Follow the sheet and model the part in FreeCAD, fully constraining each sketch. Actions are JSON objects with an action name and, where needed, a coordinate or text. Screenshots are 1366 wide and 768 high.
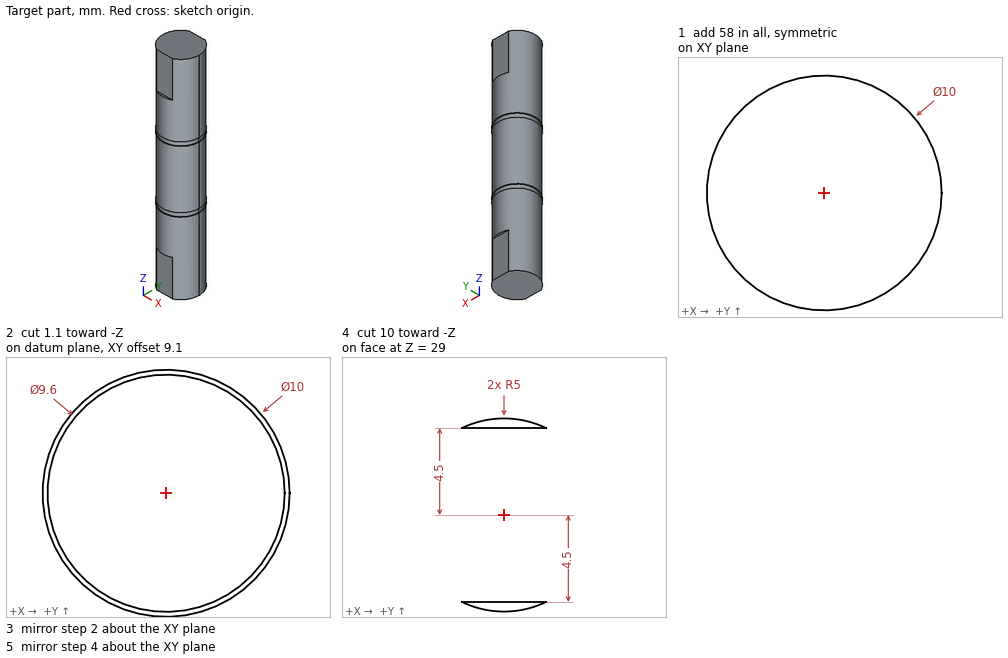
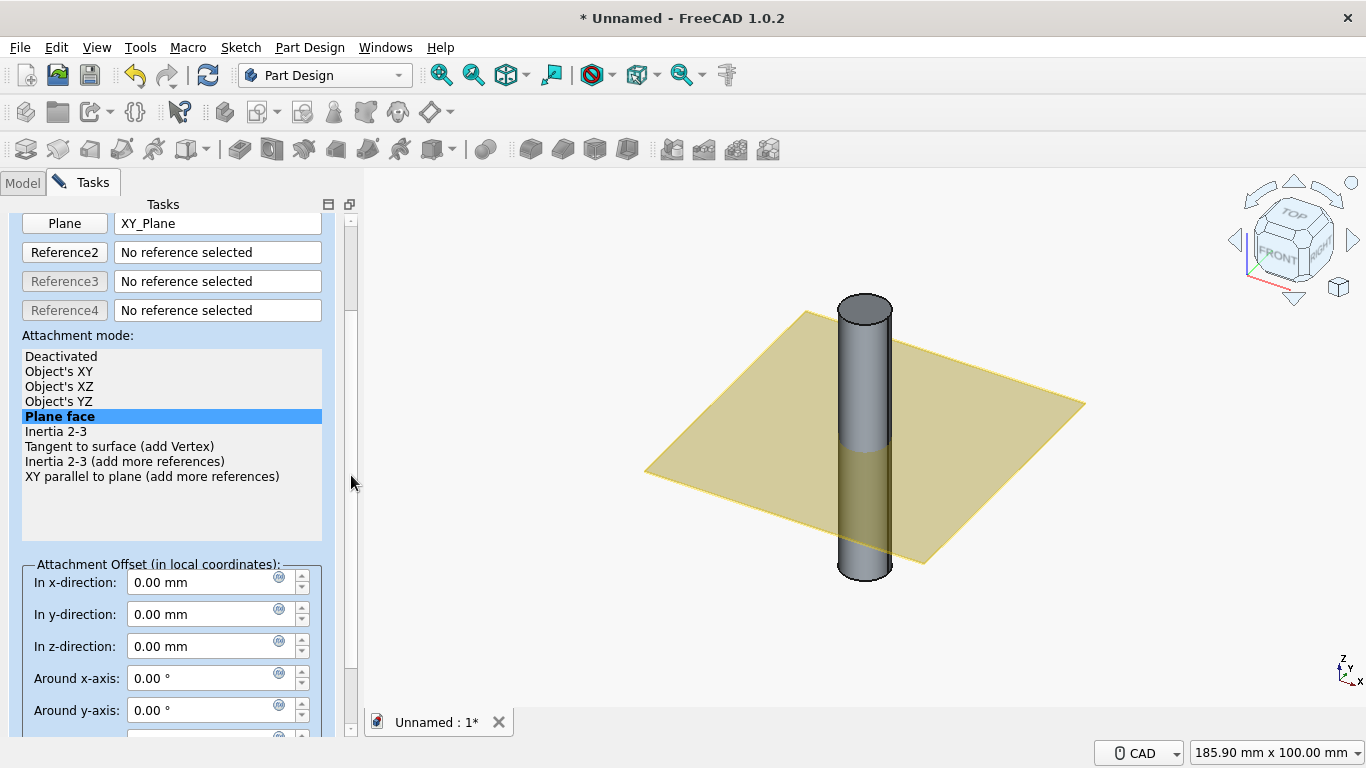
{"action": "triple_click", "coordinate": [210, 646]}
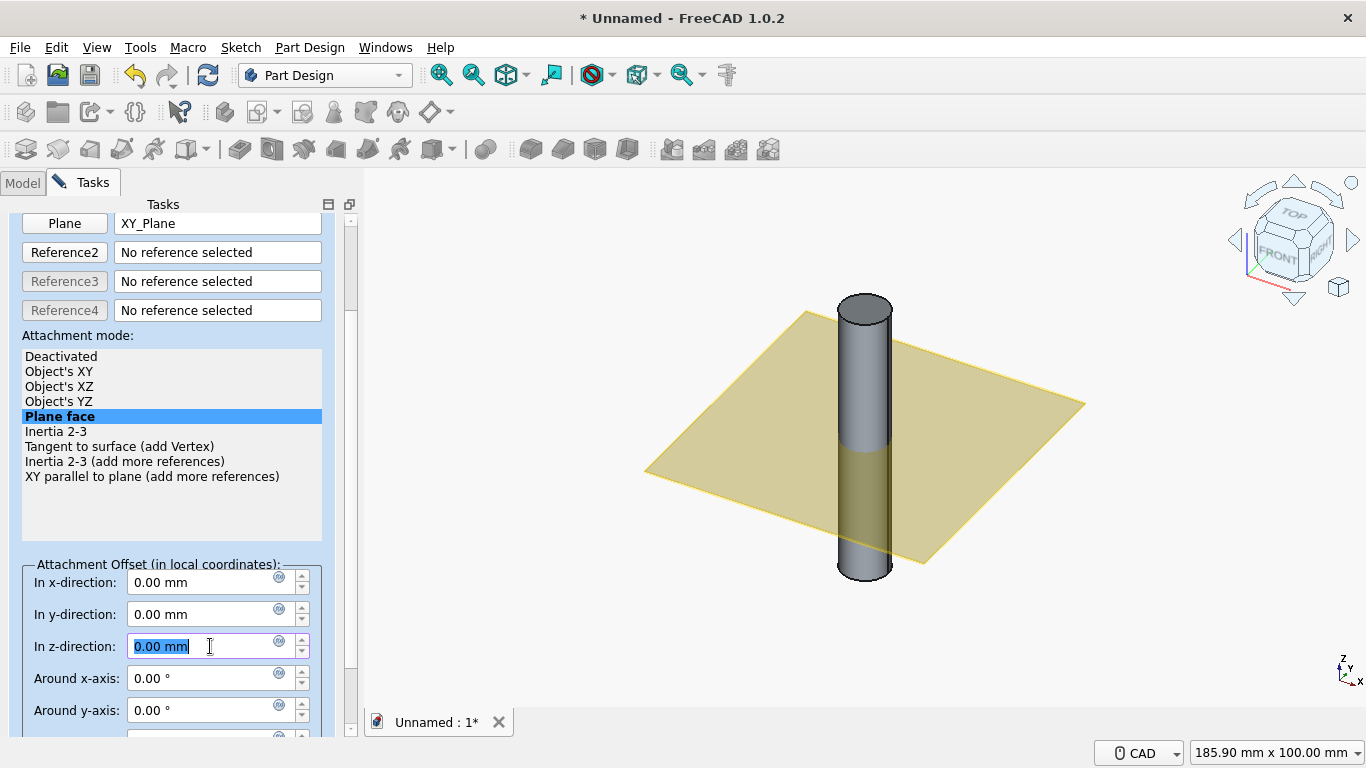
{"action": "type", "text": "9.1"}
{"action": "key", "text": "Tab"}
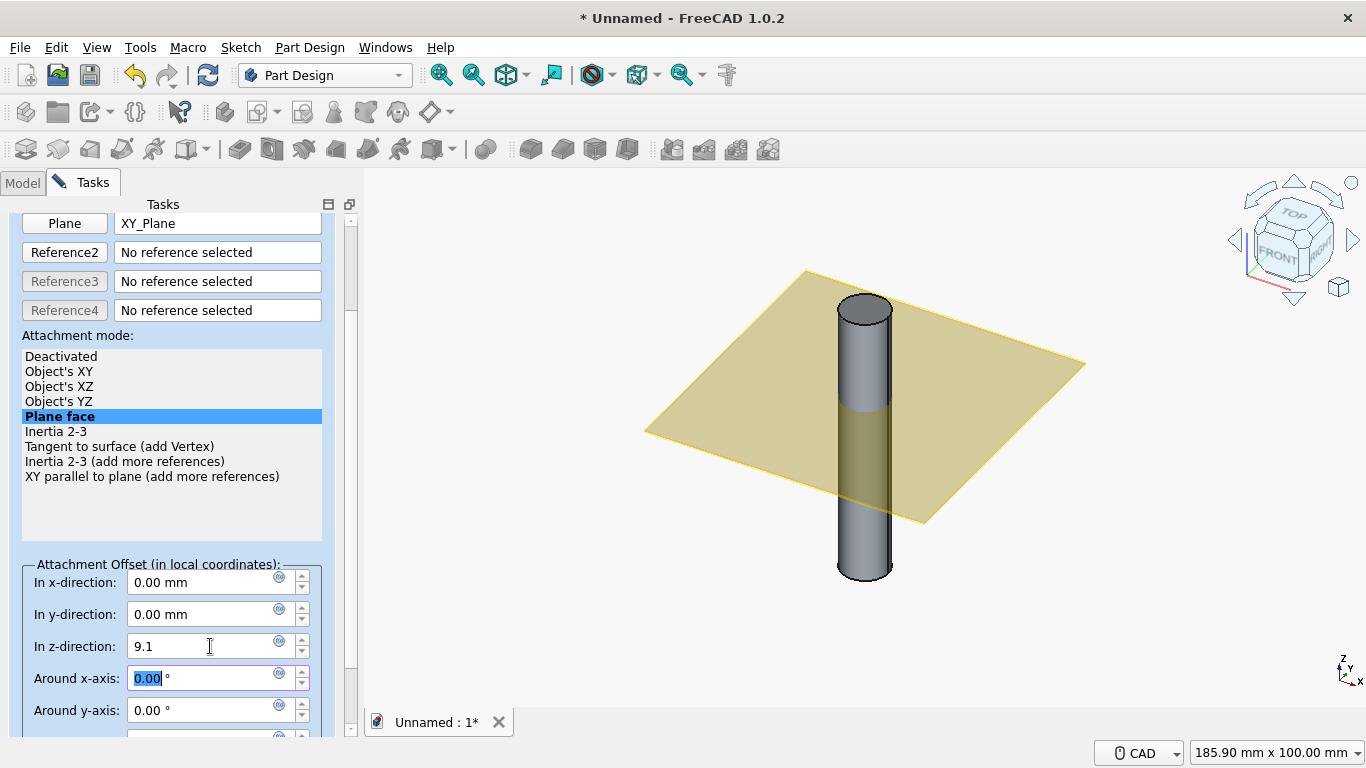
{"action": "scroll", "coordinate": [351, 475], "scroll_direction": "up", "scroll_amount": 3}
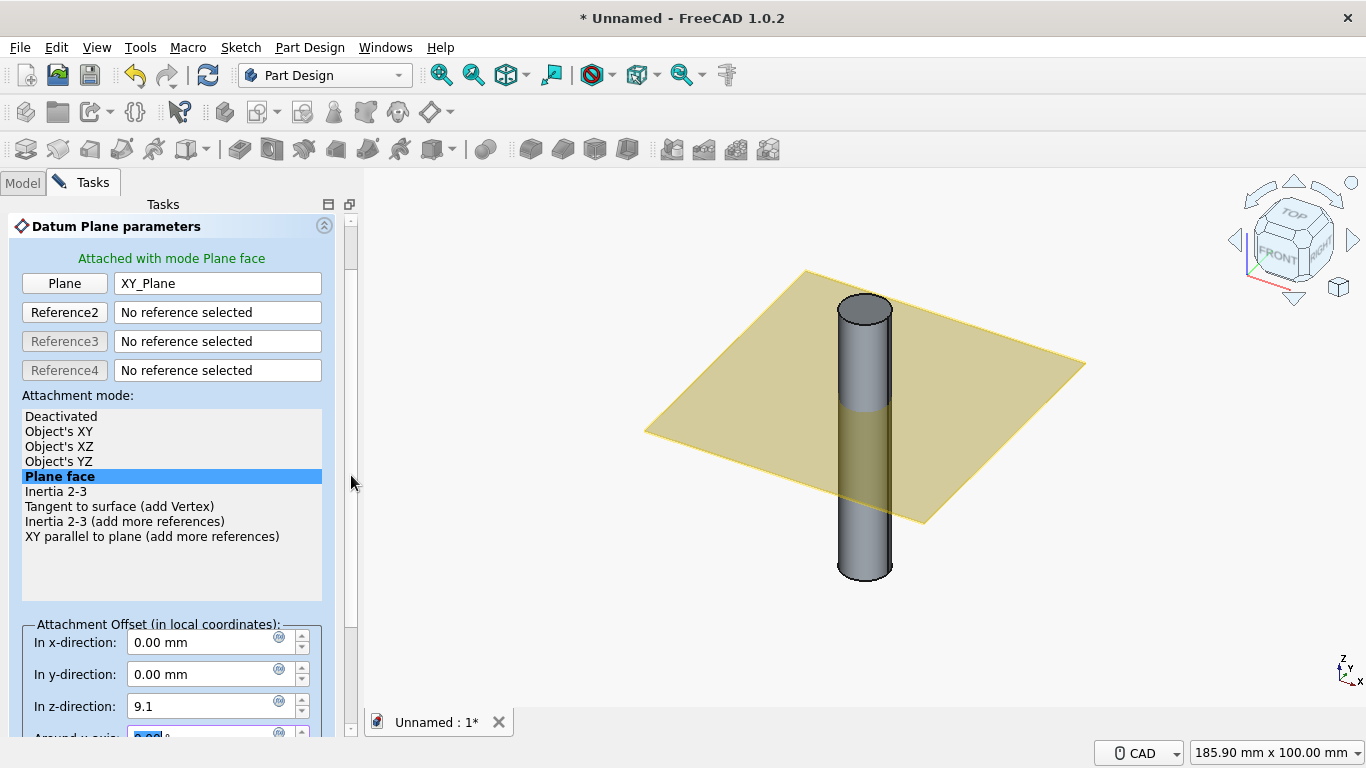
{"action": "left_click", "coordinate": [124, 243]}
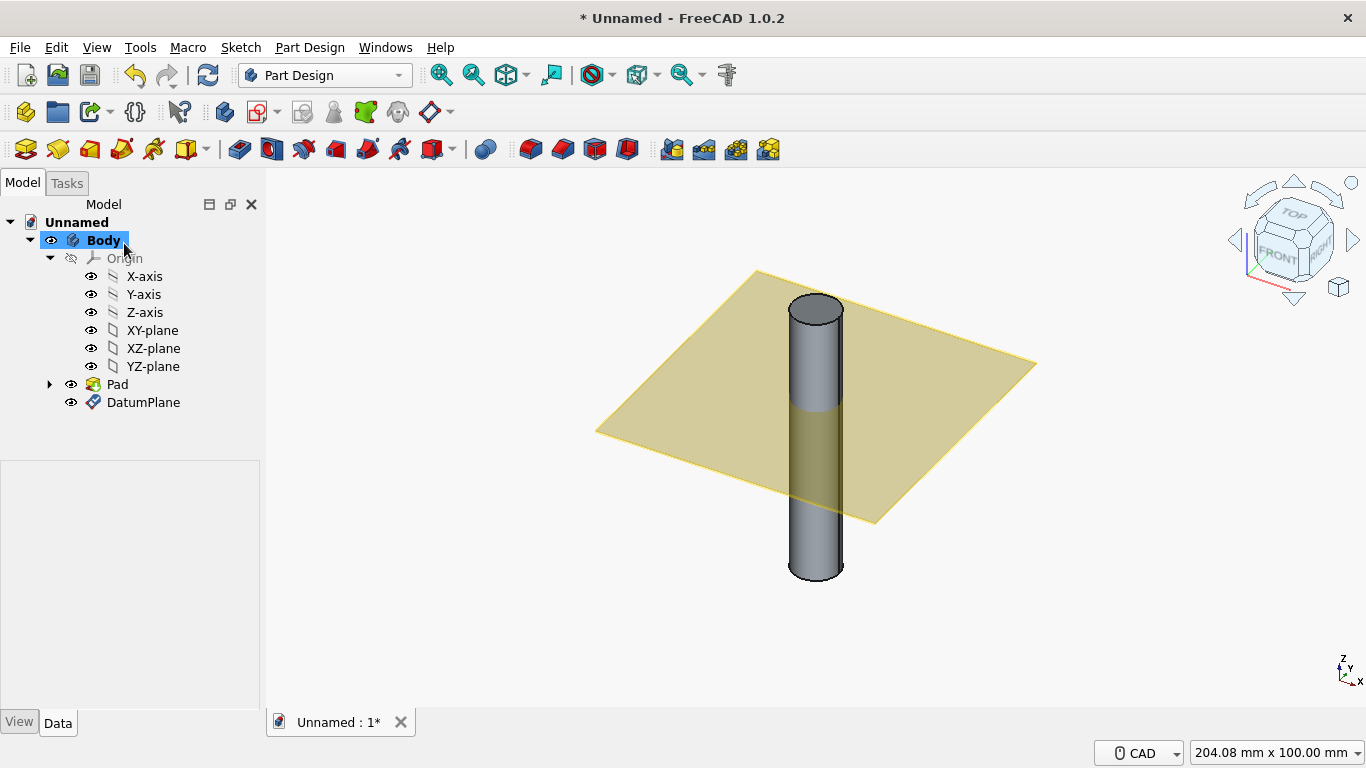
{"action": "left_click", "coordinate": [116, 402]}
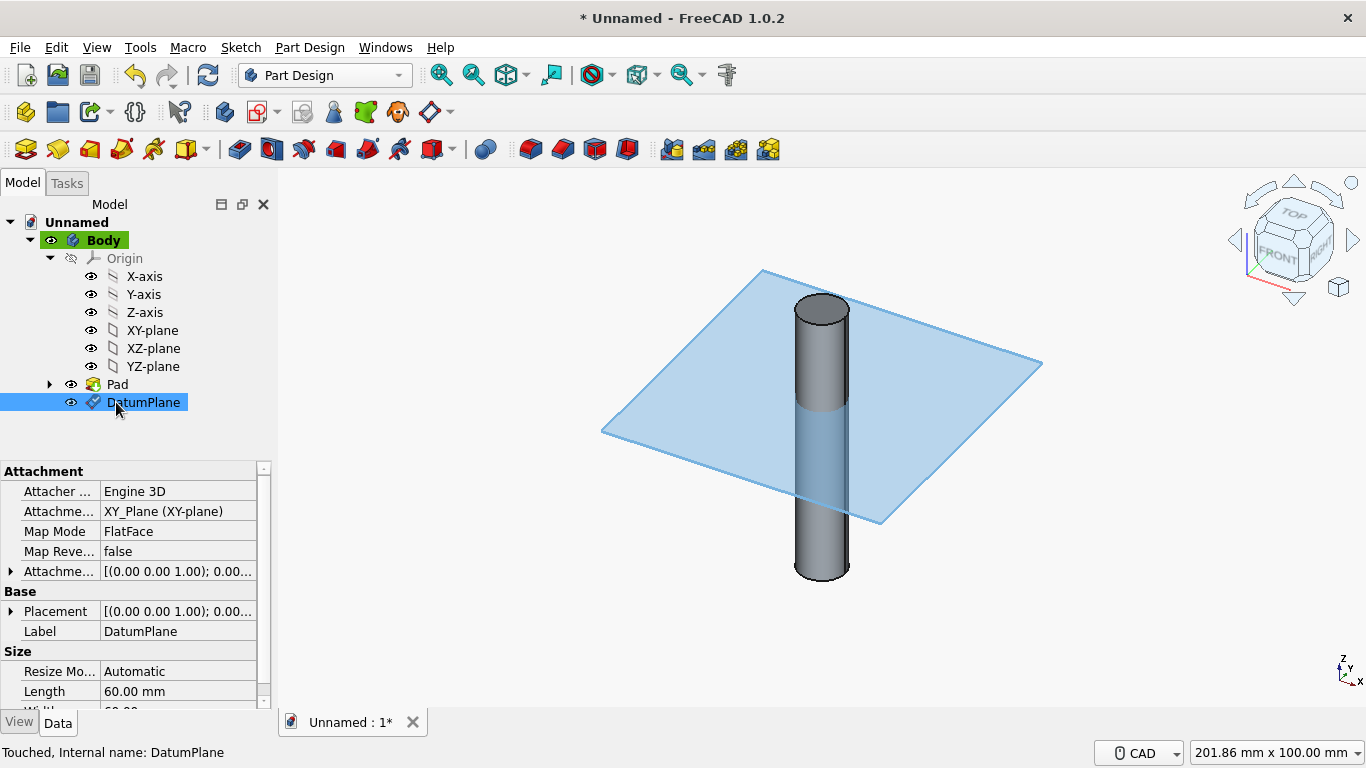
{"action": "left_click", "coordinate": [258, 112]}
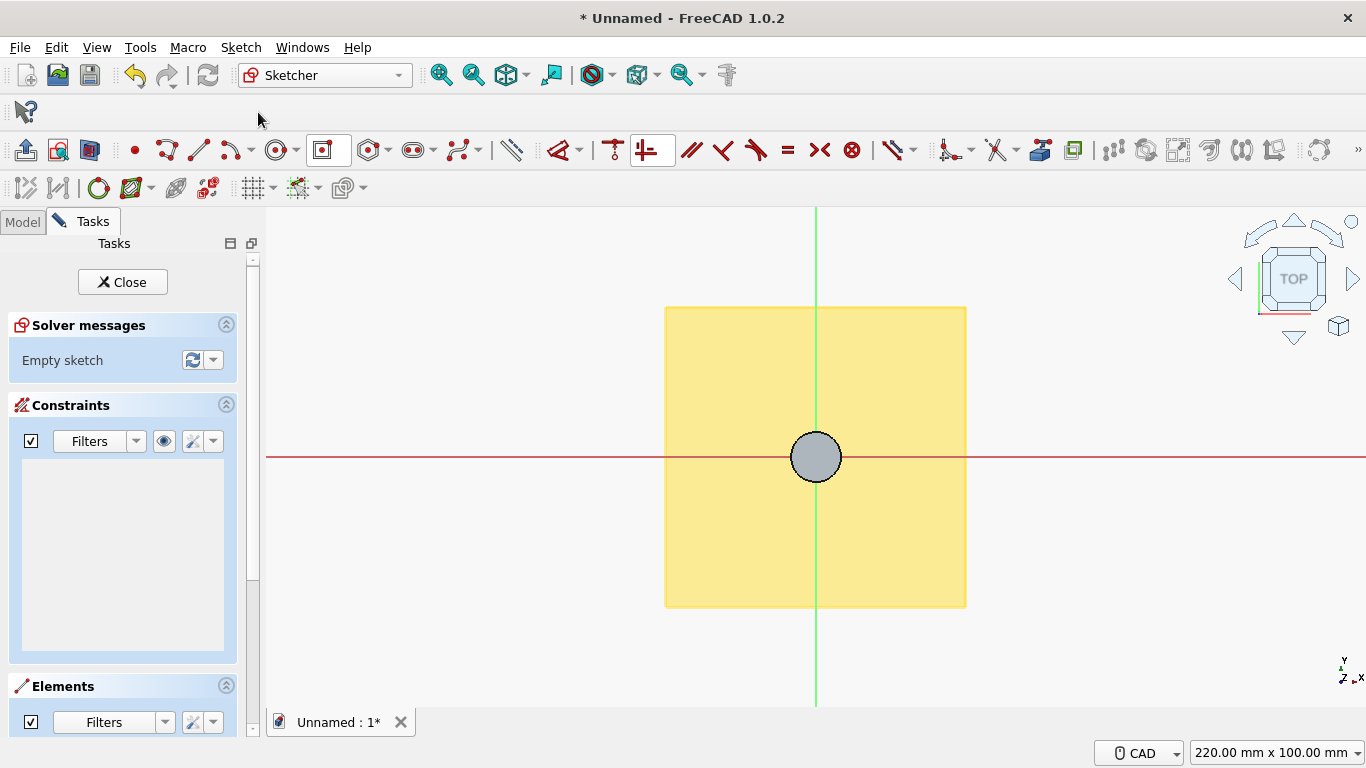
{"action": "left_click", "coordinate": [90, 150]}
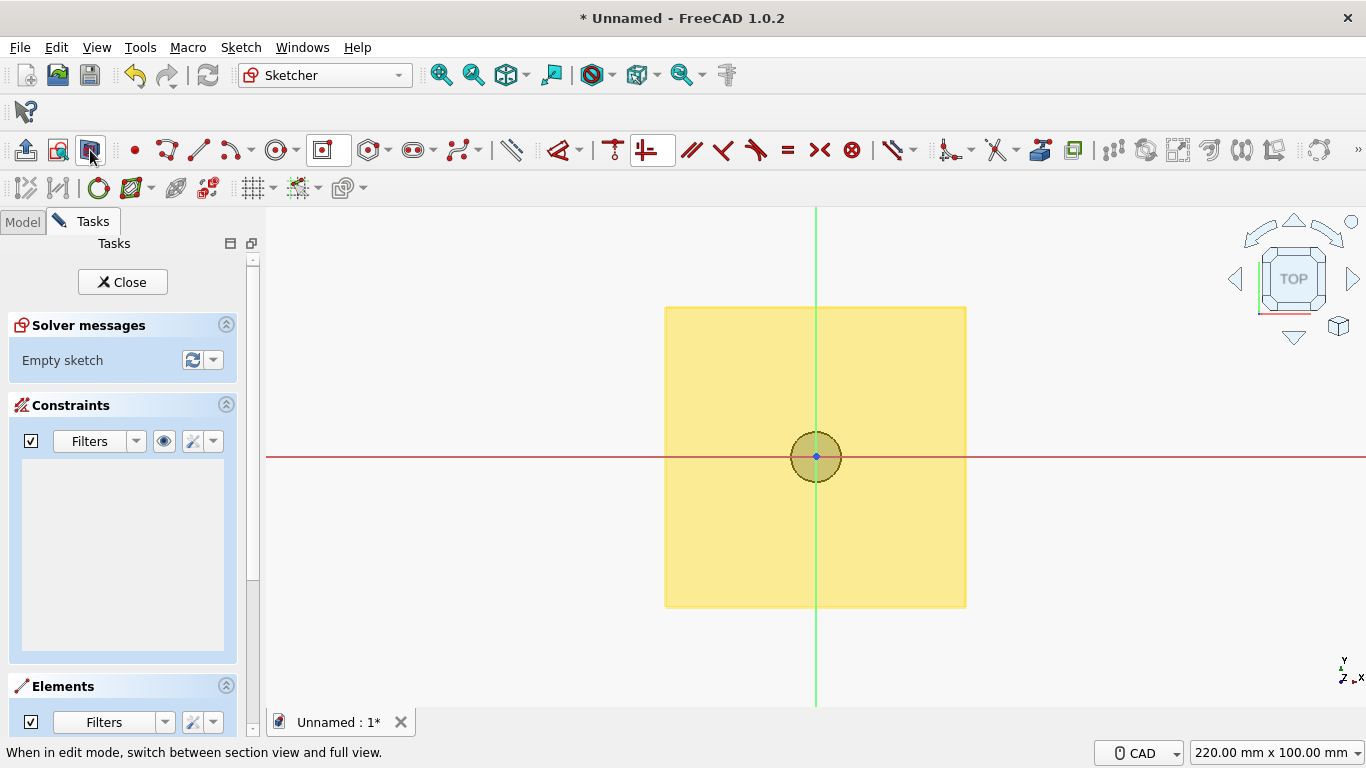
{"action": "scroll", "coordinate": [830, 457], "scroll_direction": "up", "scroll_amount": 9}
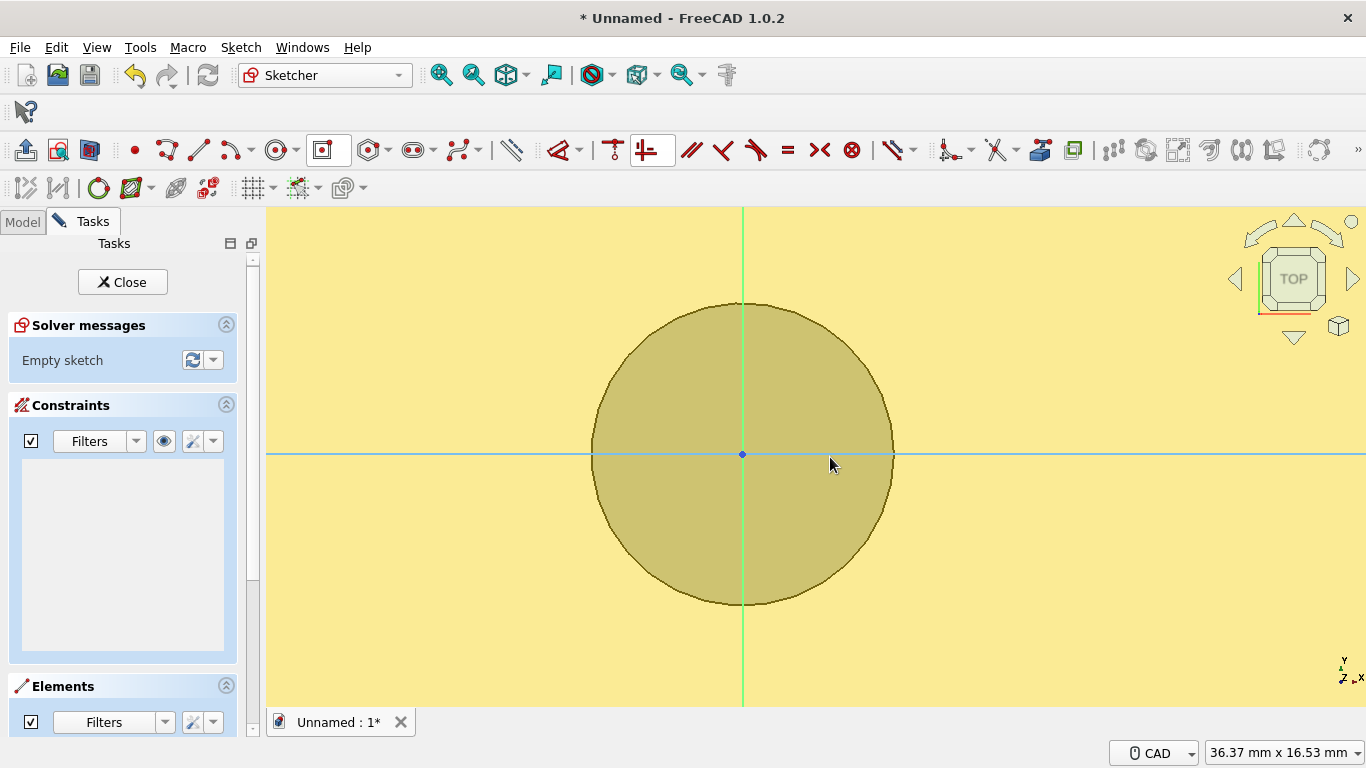
{"action": "left_click", "coordinate": [276, 150]}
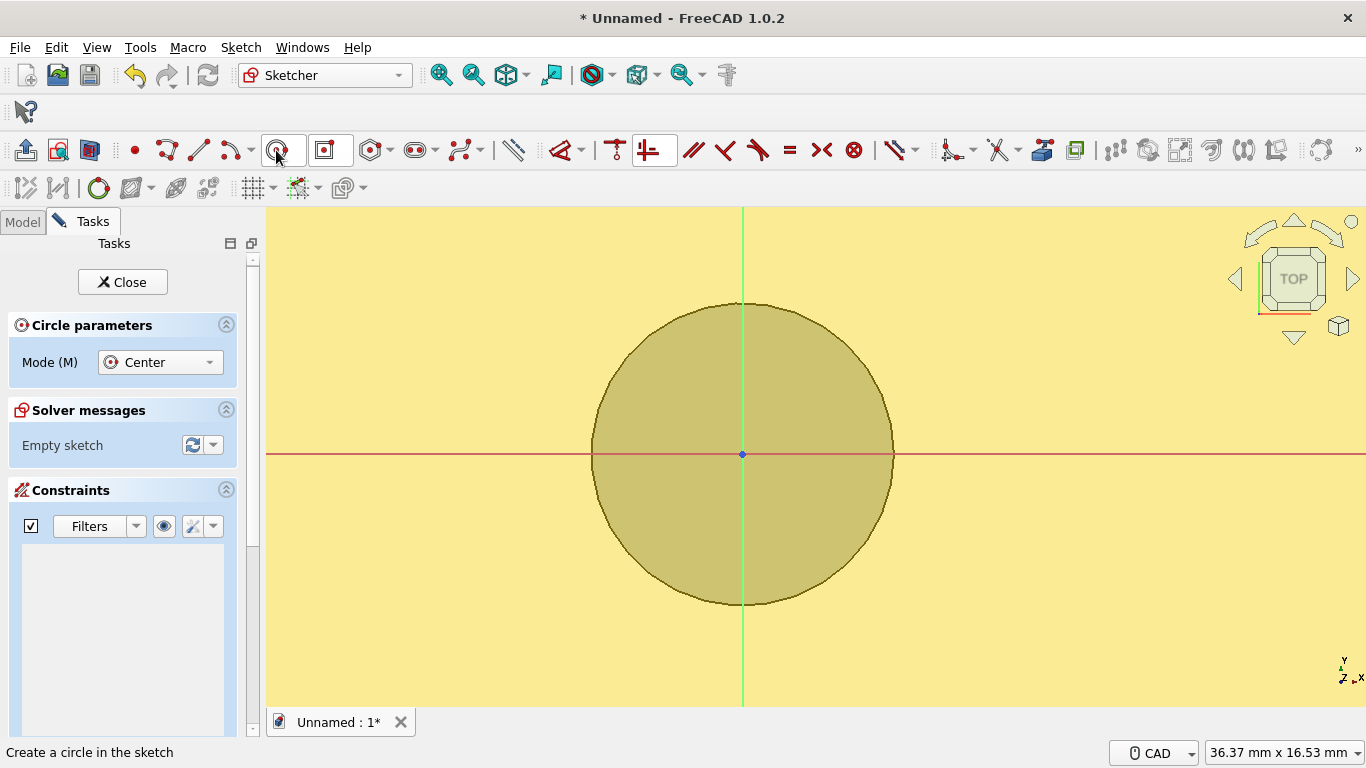
{"action": "left_click", "coordinate": [743, 454]}
{"action": "left_click", "coordinate": [850, 348]}